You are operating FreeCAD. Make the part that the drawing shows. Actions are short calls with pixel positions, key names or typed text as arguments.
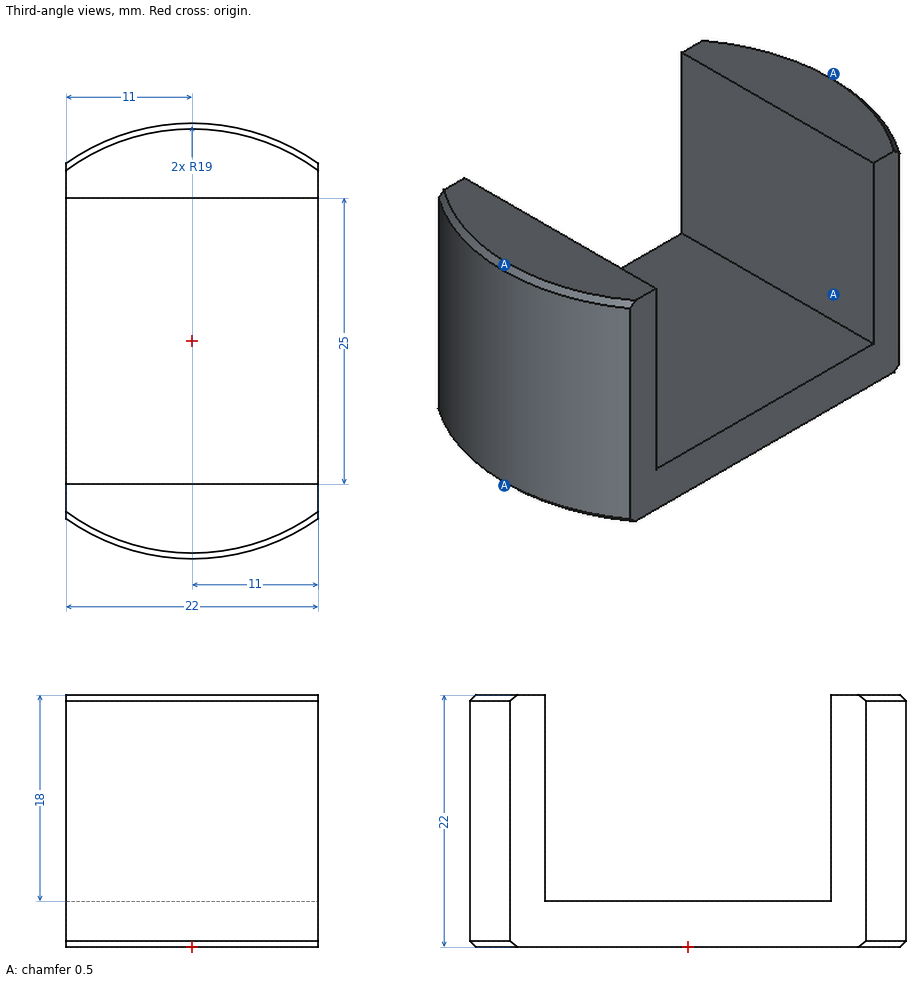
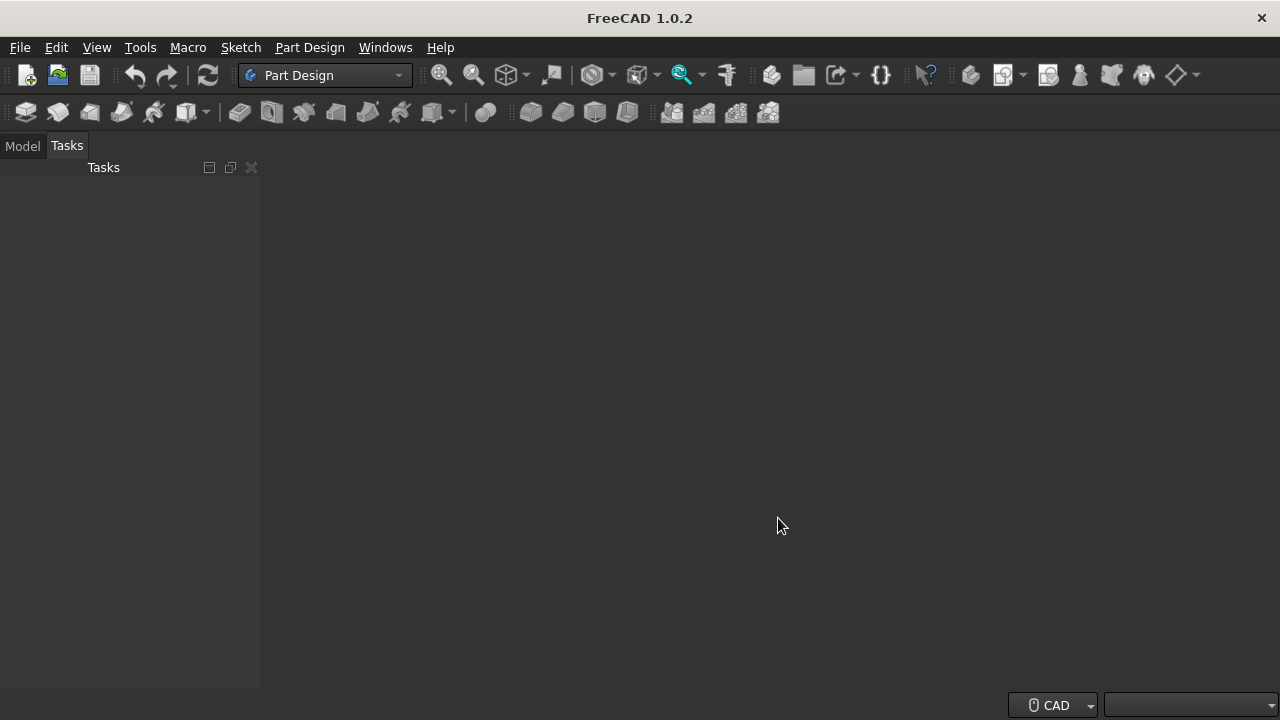
click(26, 76)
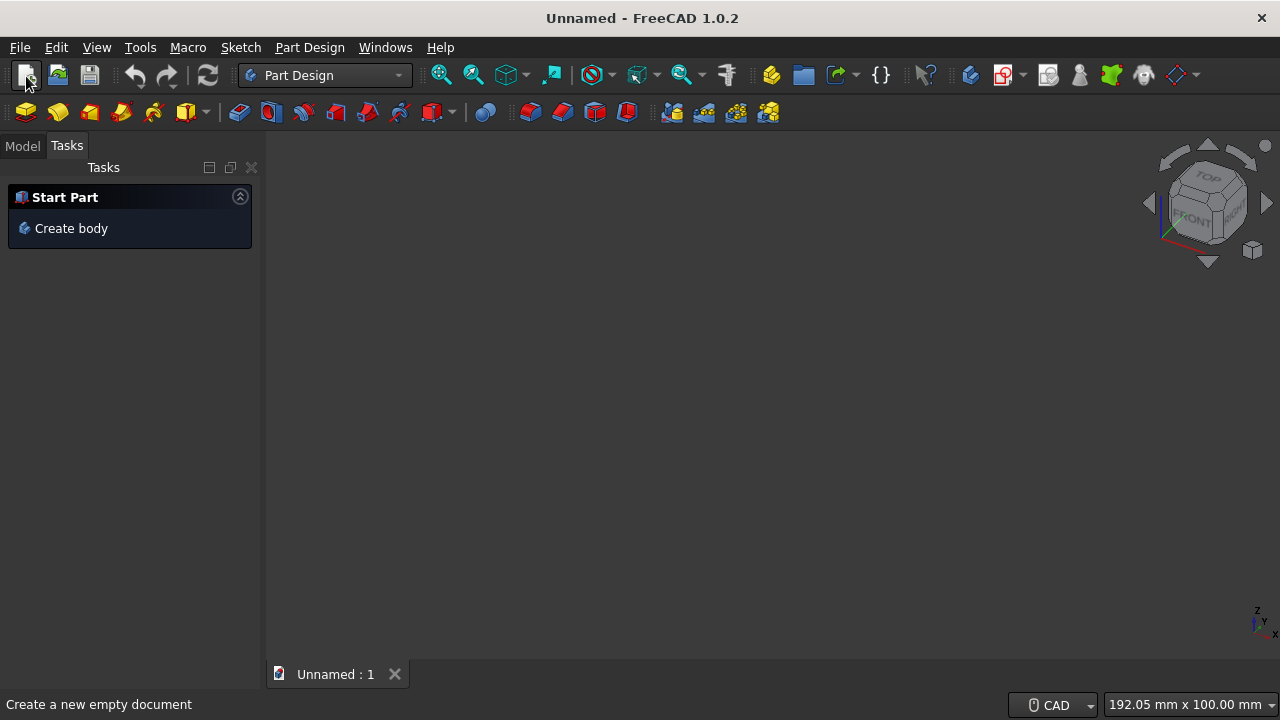
click(1004, 76)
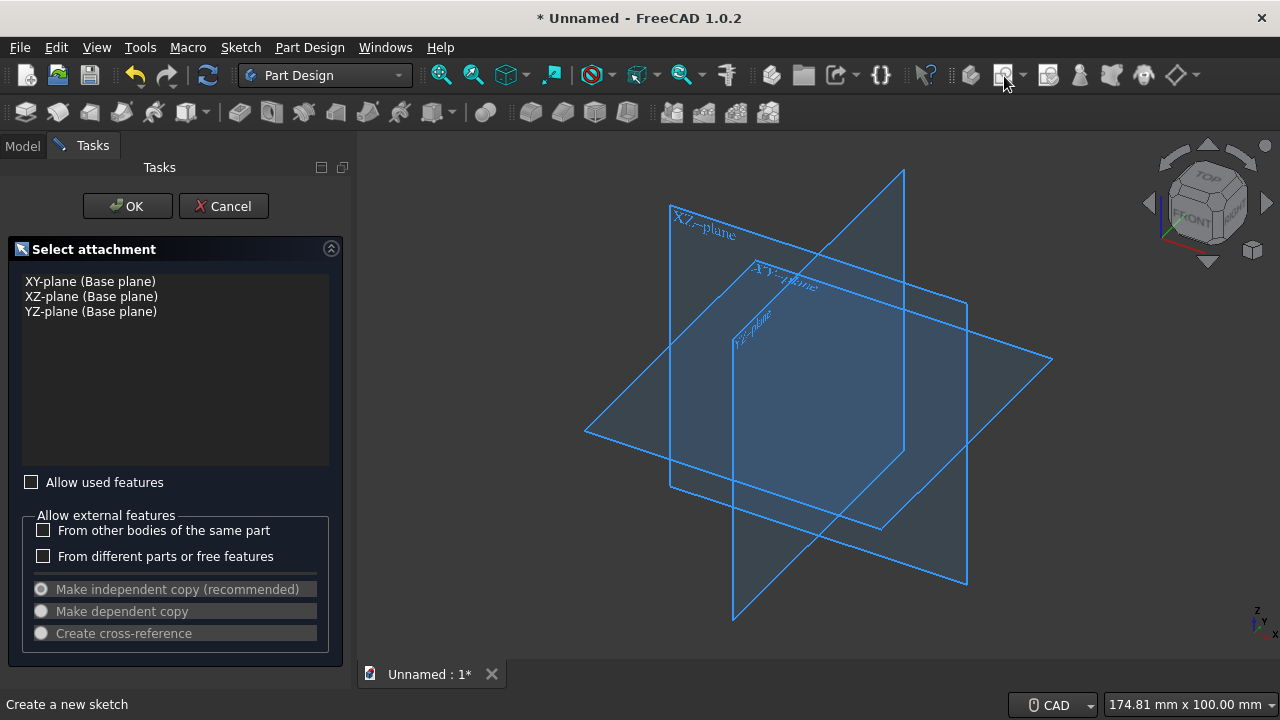
click(82, 282)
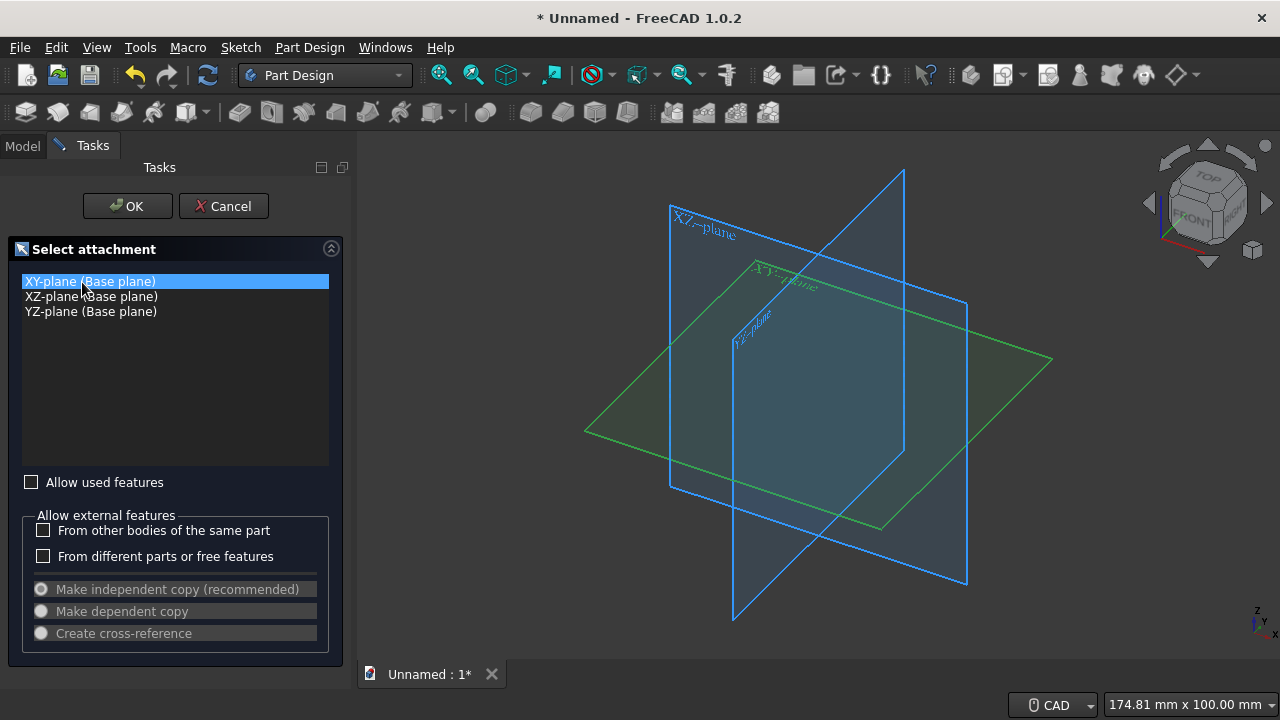
click(128, 206)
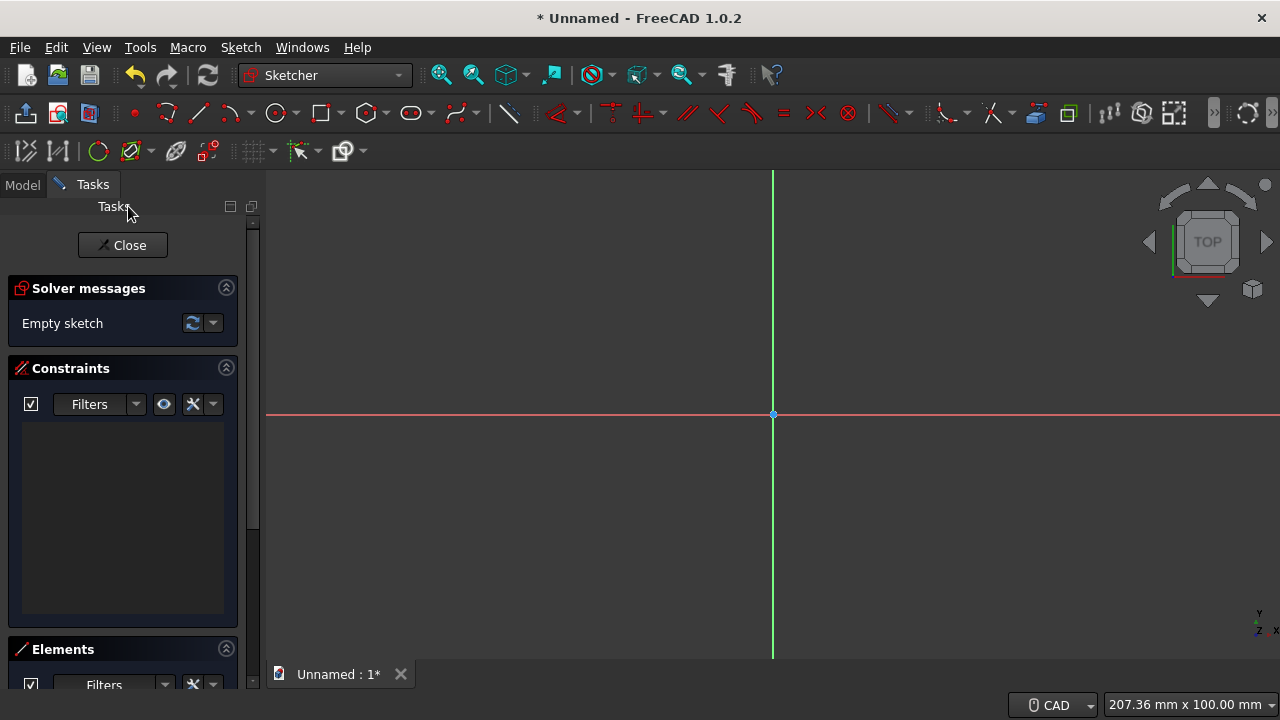
scroll(912, 414, up, 2)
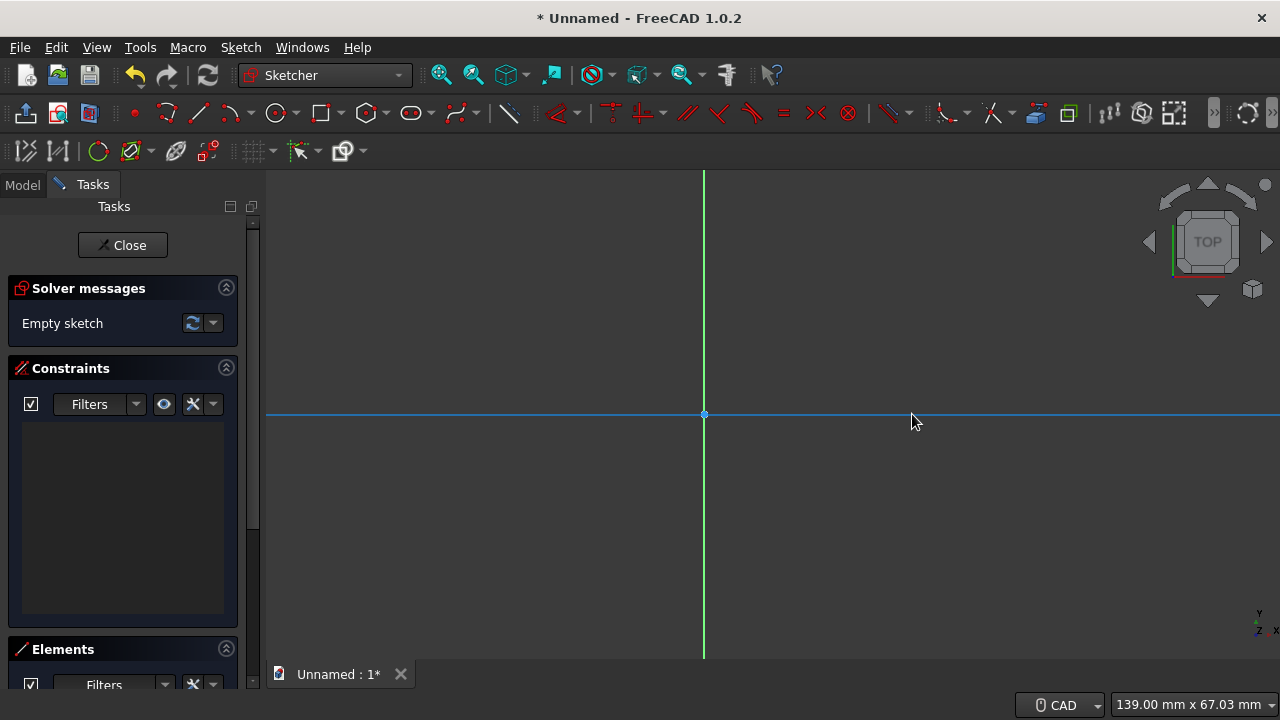
click(200, 114)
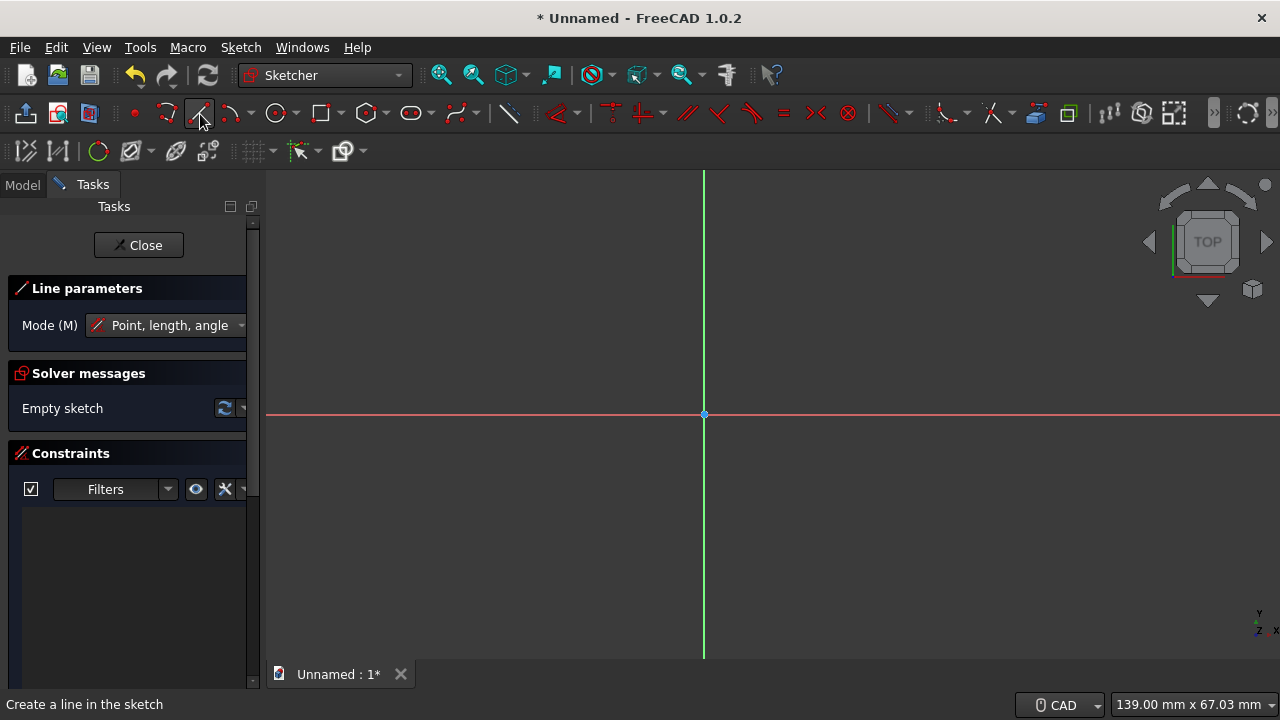
click(785, 528)
click(785, 301)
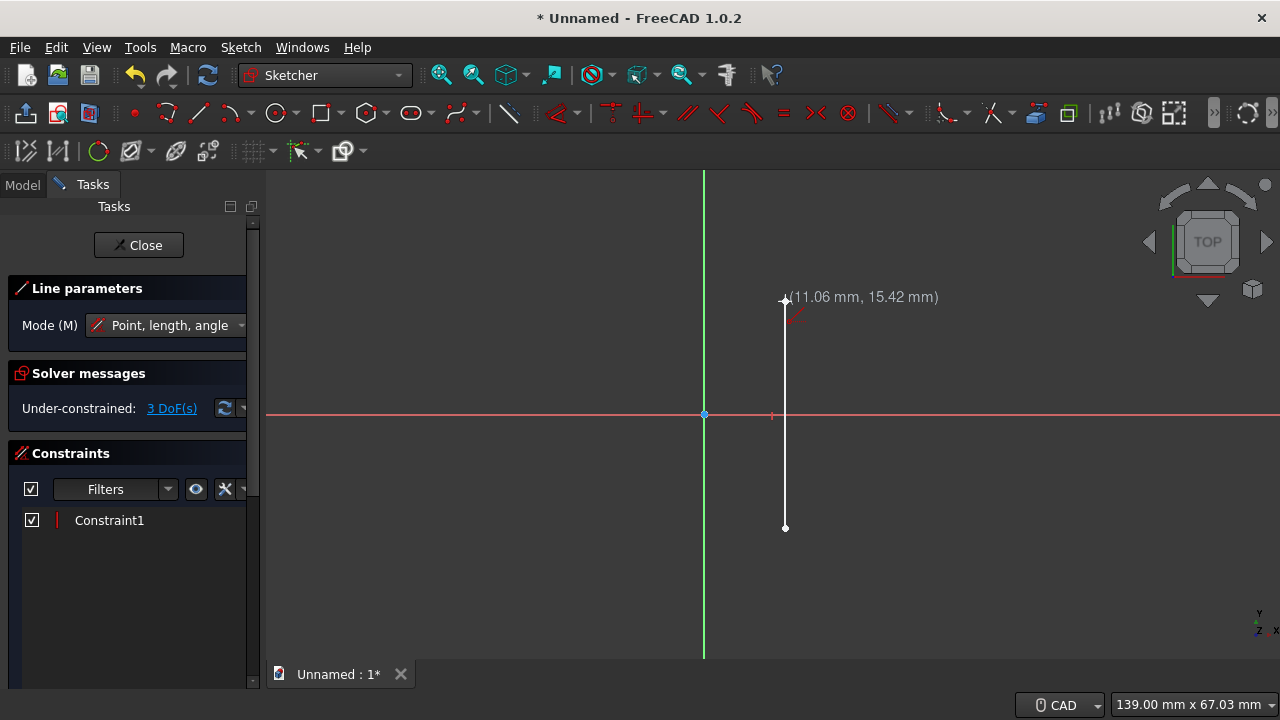
click(624, 301)
click(624, 528)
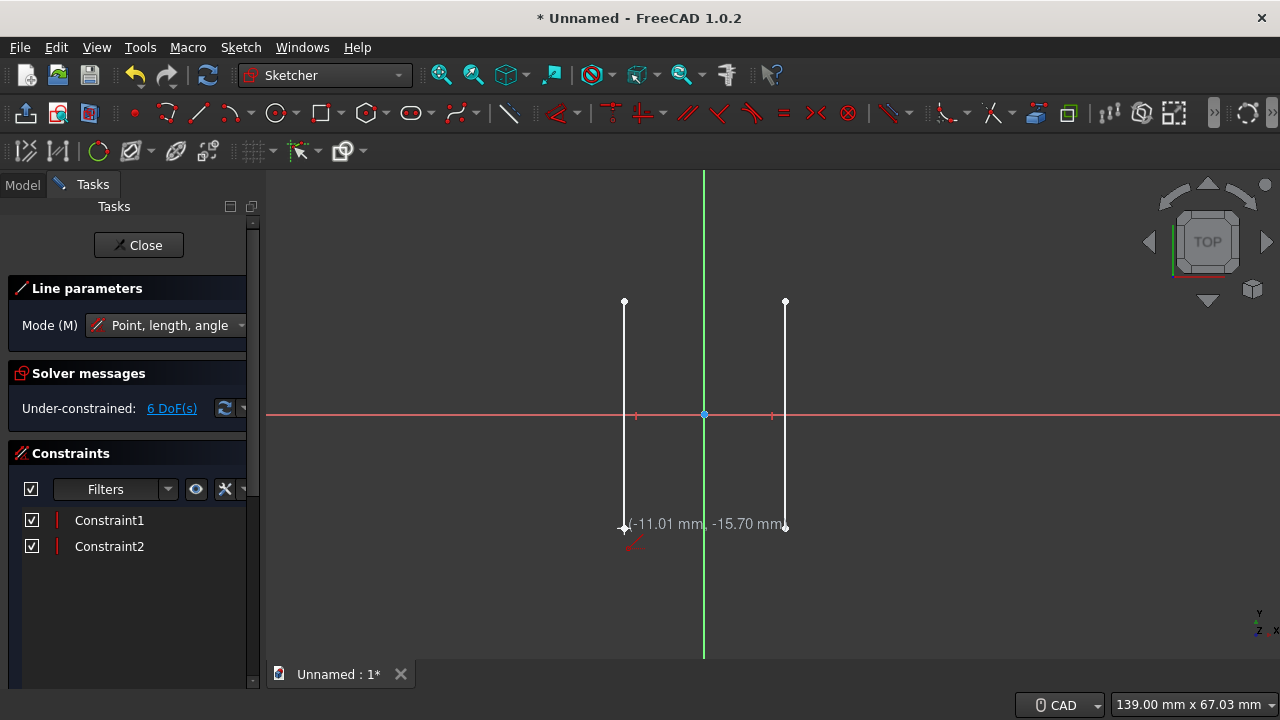
key(g)
key(3)
key(a)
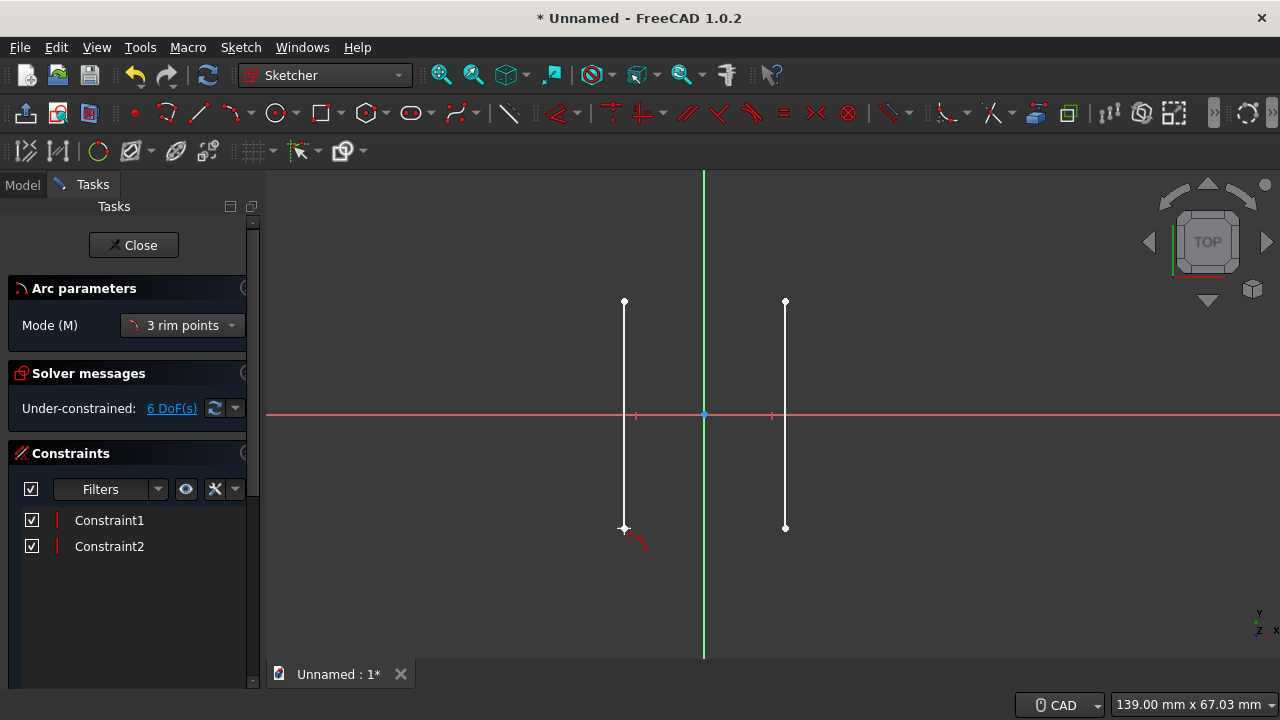
click(785, 302)
click(624, 302)
click(721, 277)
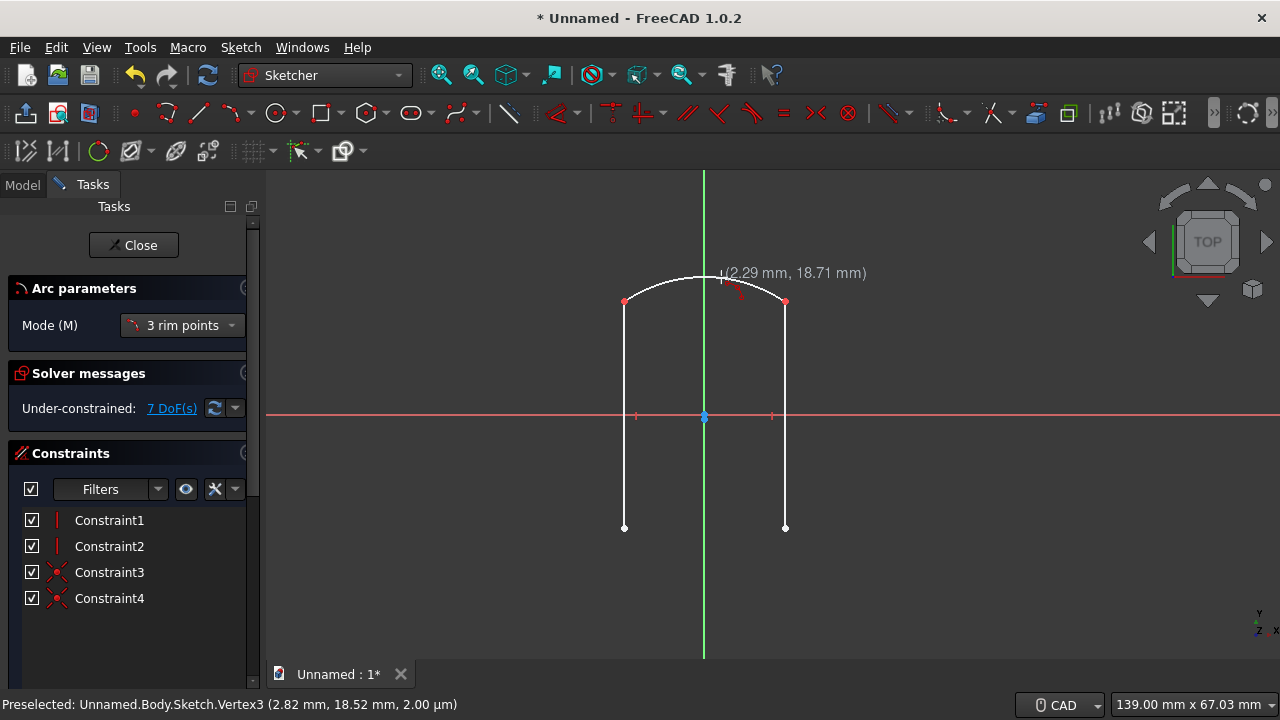
click(624, 529)
click(785, 529)
click(687, 552)
key(Escape)